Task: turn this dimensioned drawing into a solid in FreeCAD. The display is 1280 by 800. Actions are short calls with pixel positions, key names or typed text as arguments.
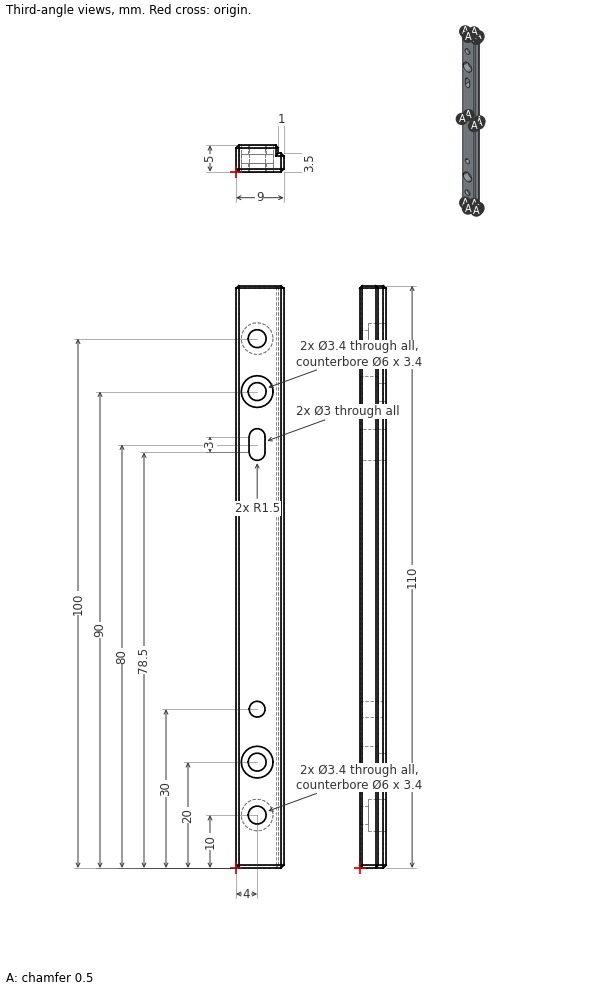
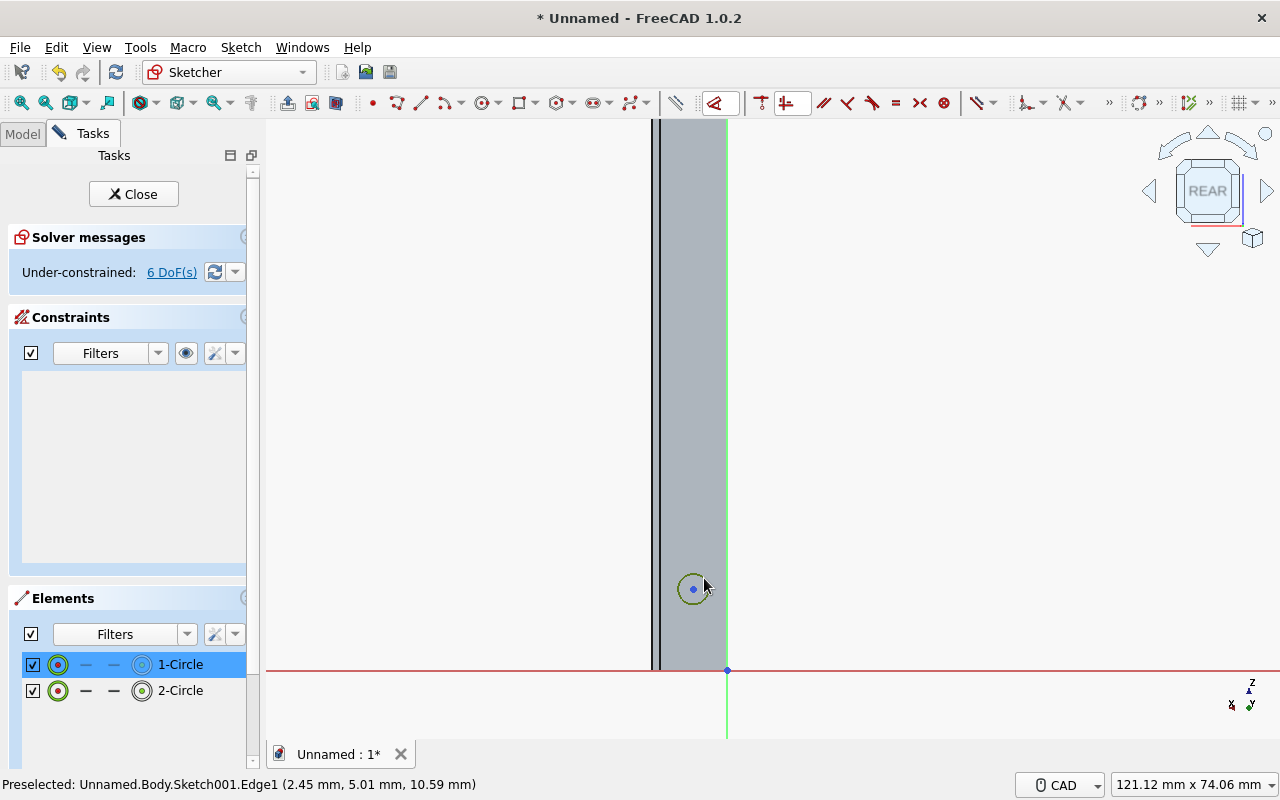
scroll(706, 579, down, 4)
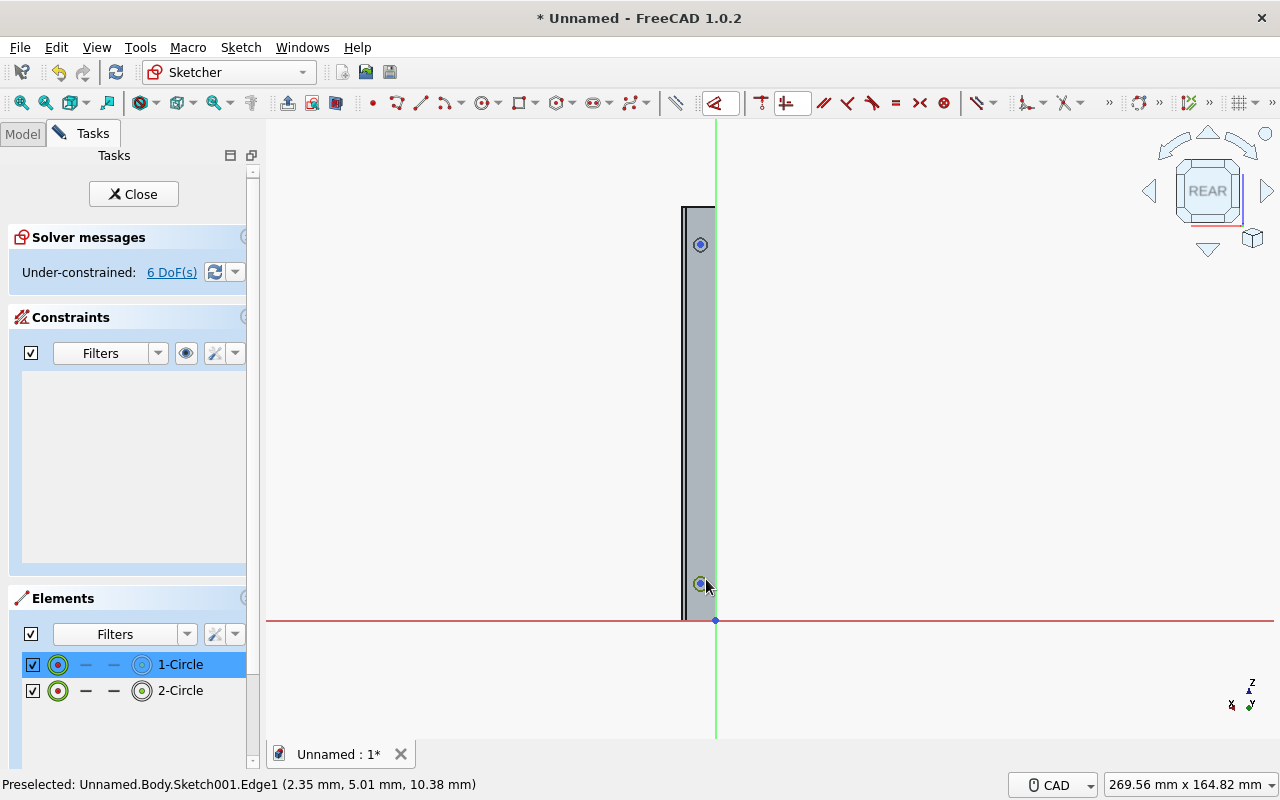
scroll(705, 240, up, 4)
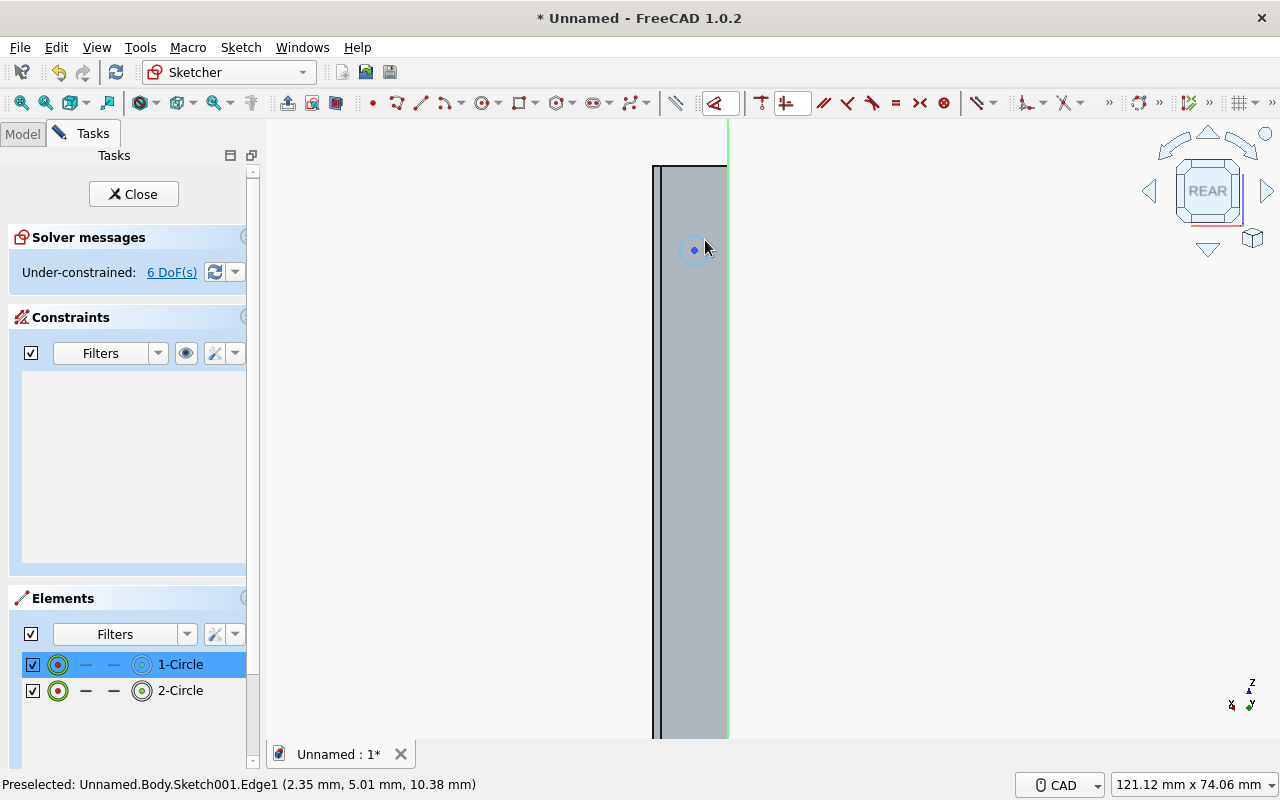
click(705, 240)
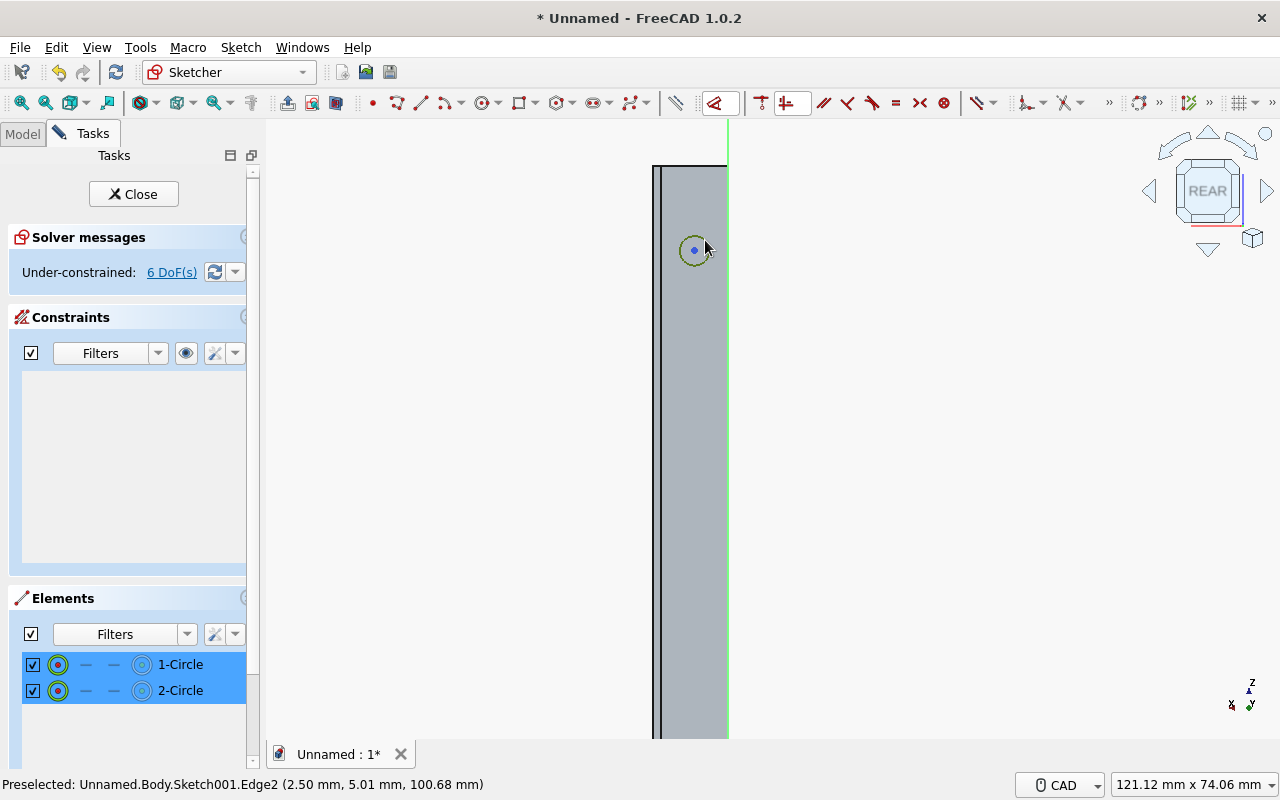
key(e)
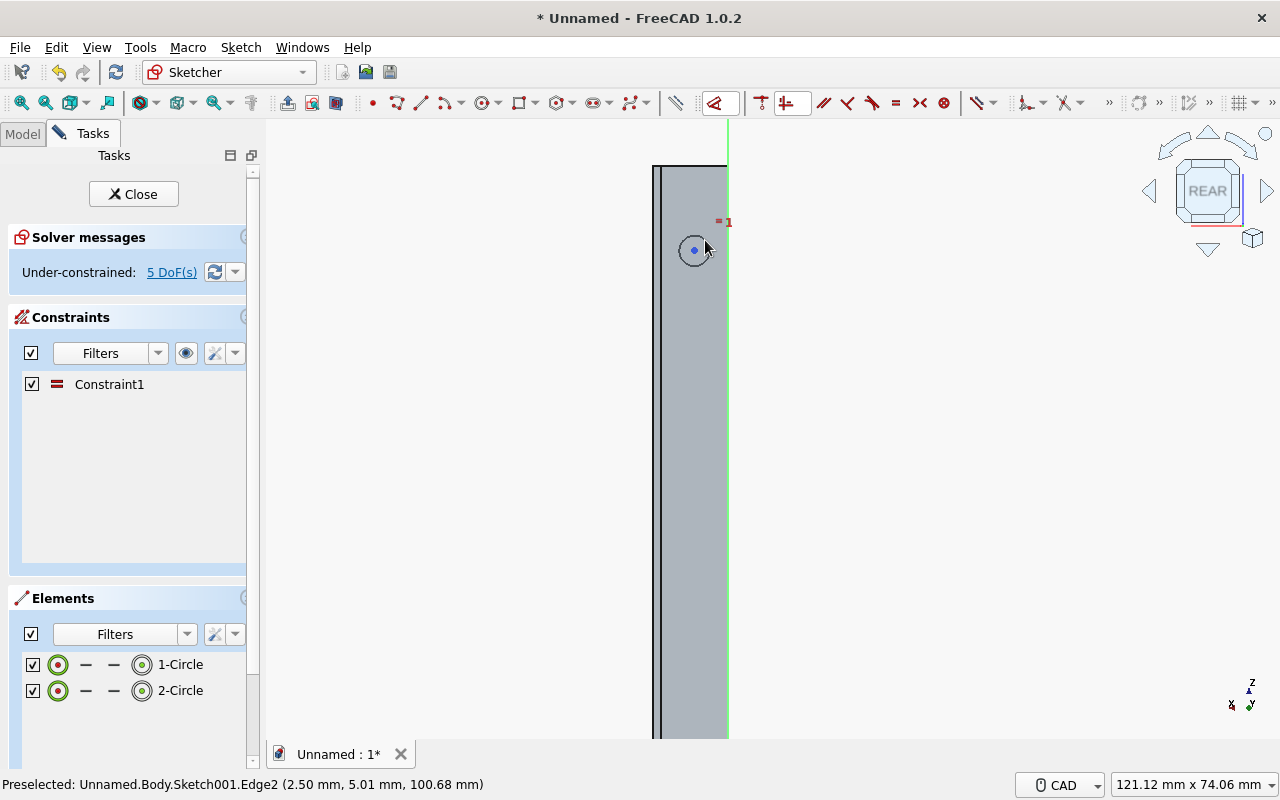
key(d)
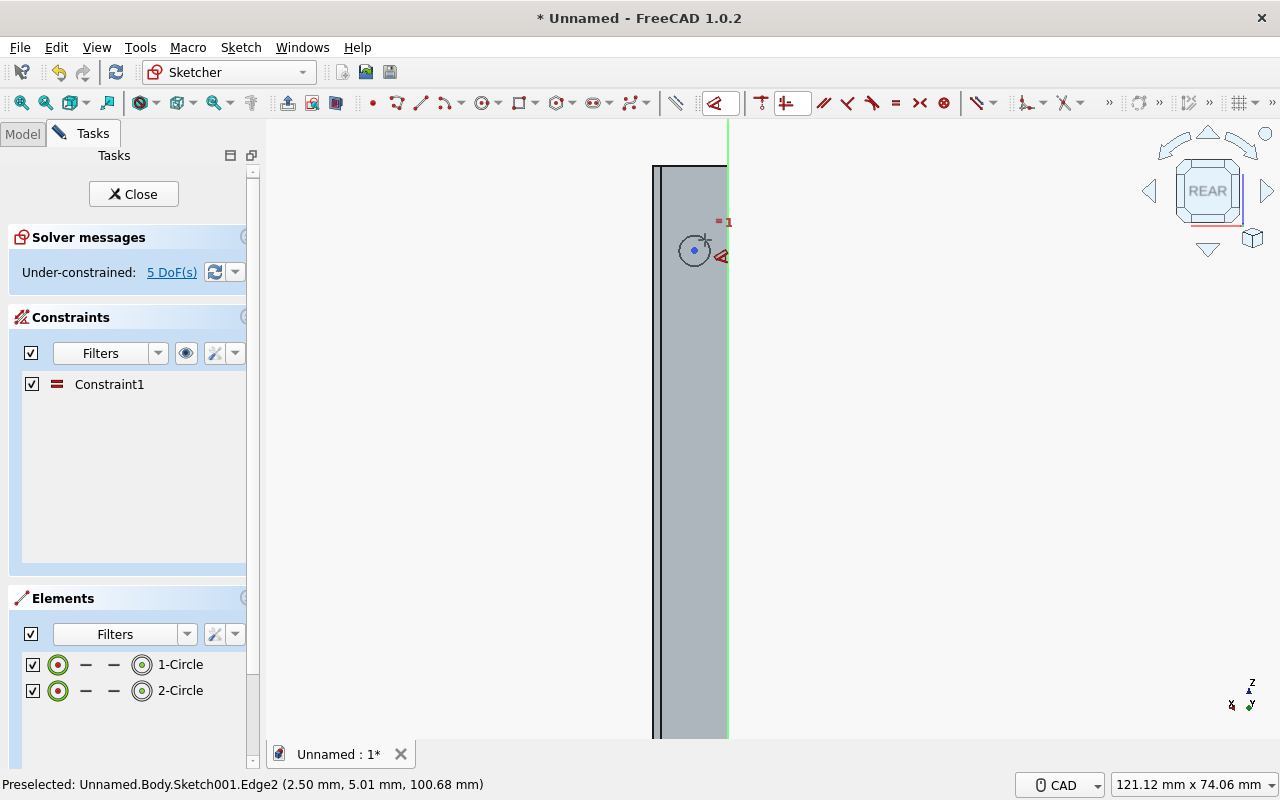
scroll(705, 240, down, 4)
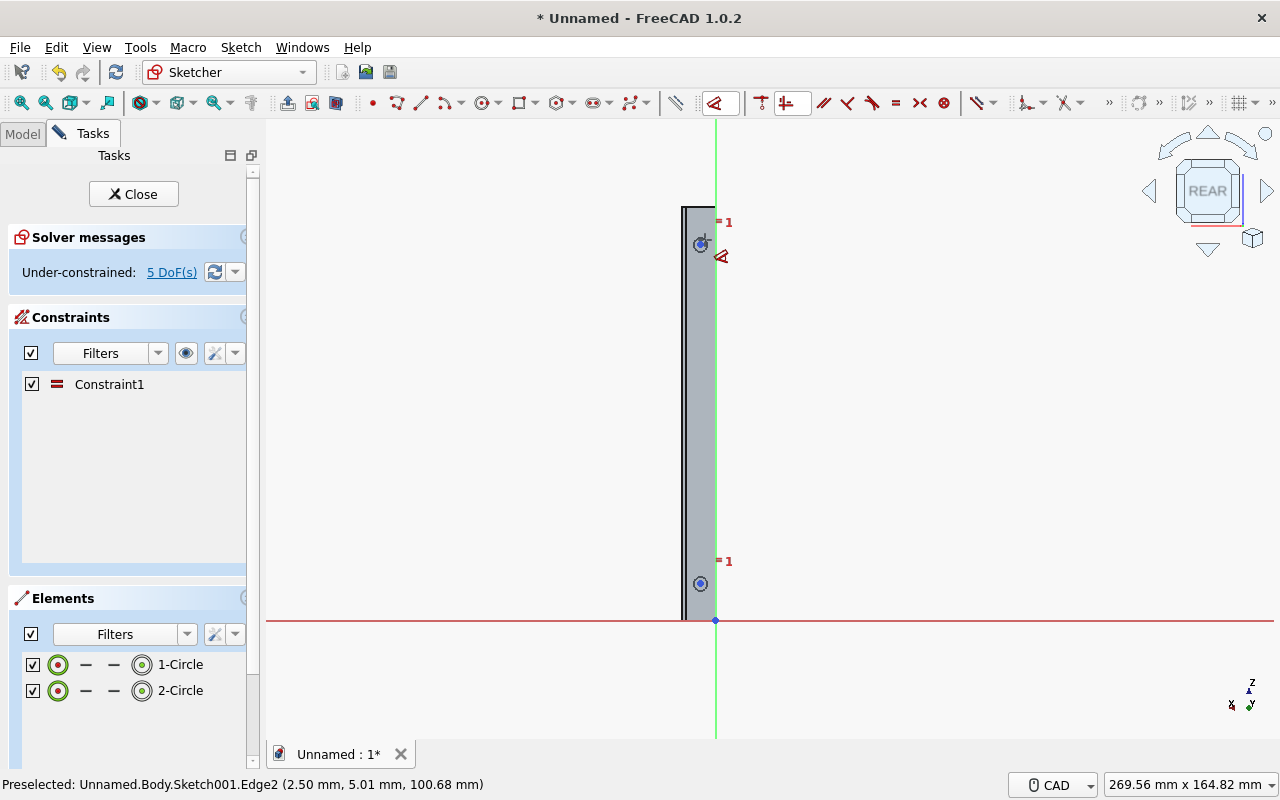
scroll(705, 579, up, 6)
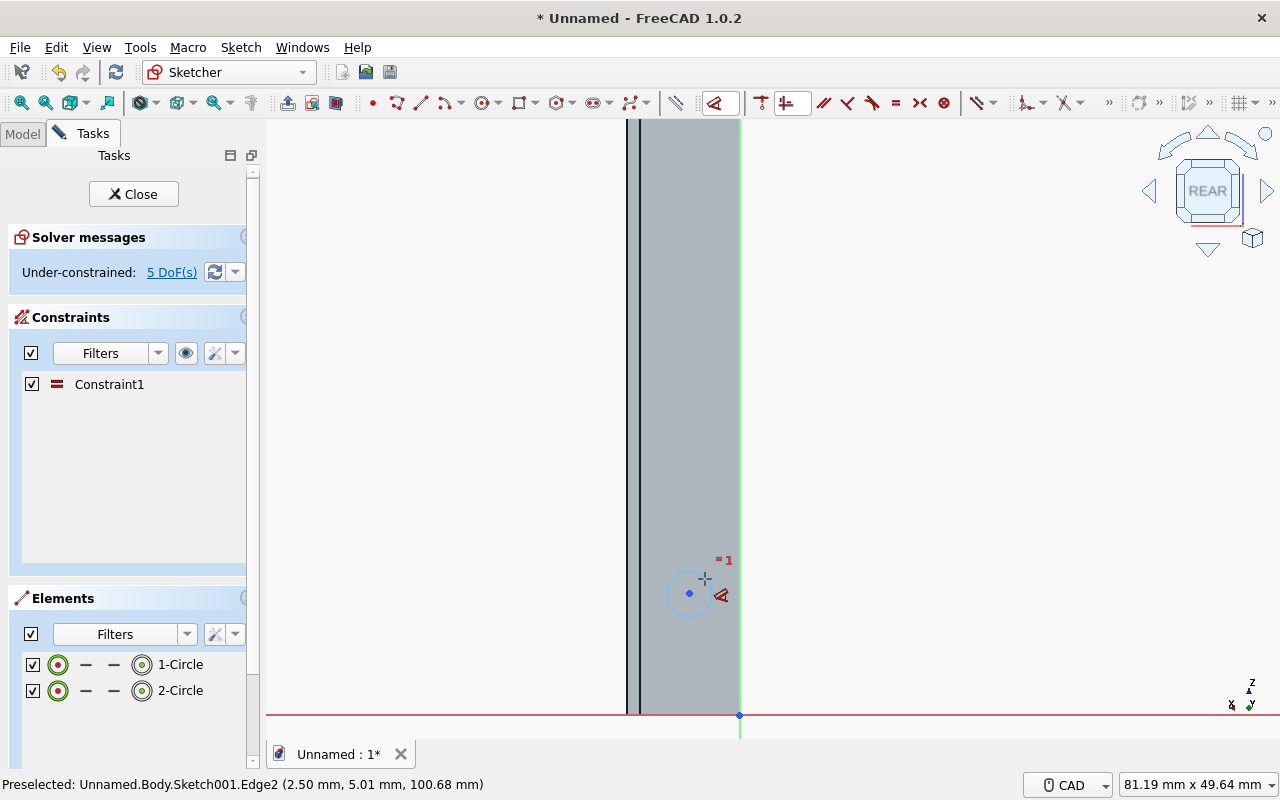
click(705, 578)
click(704, 542)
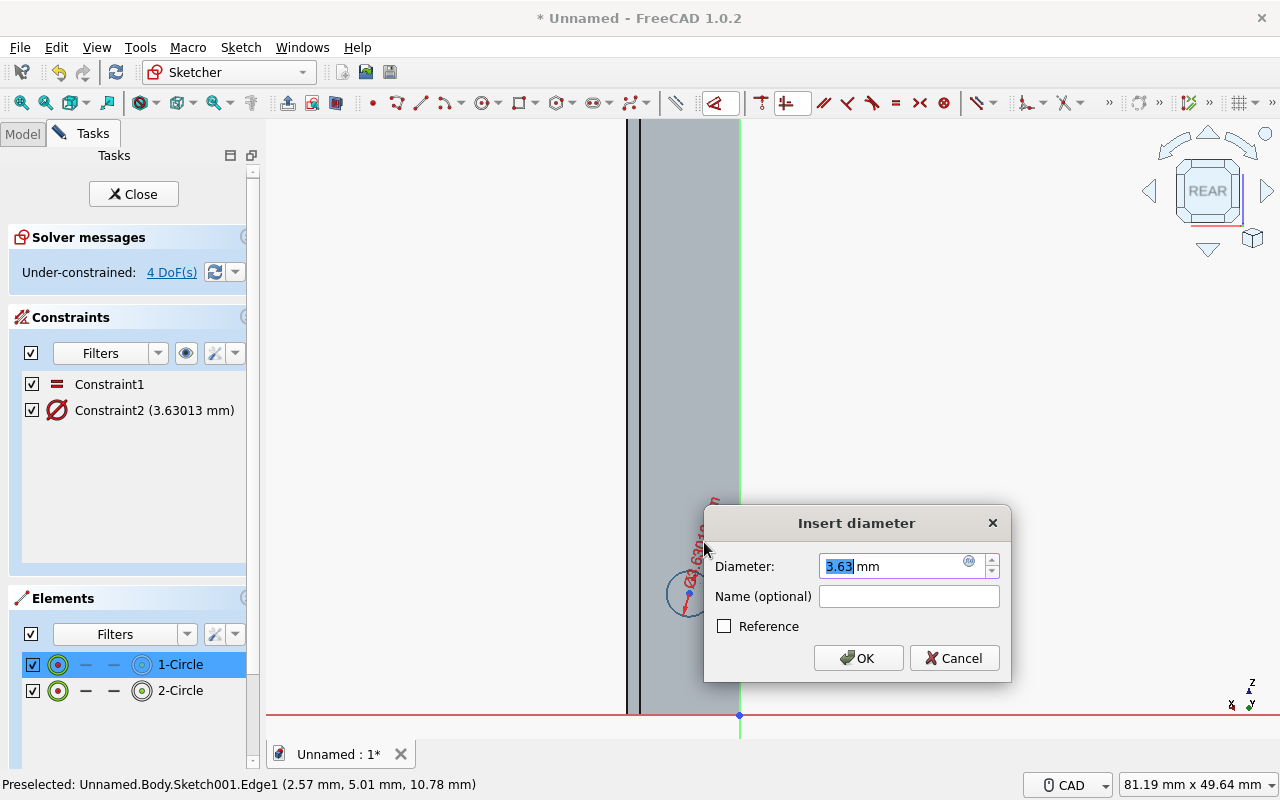
text(3.4)
key(Return)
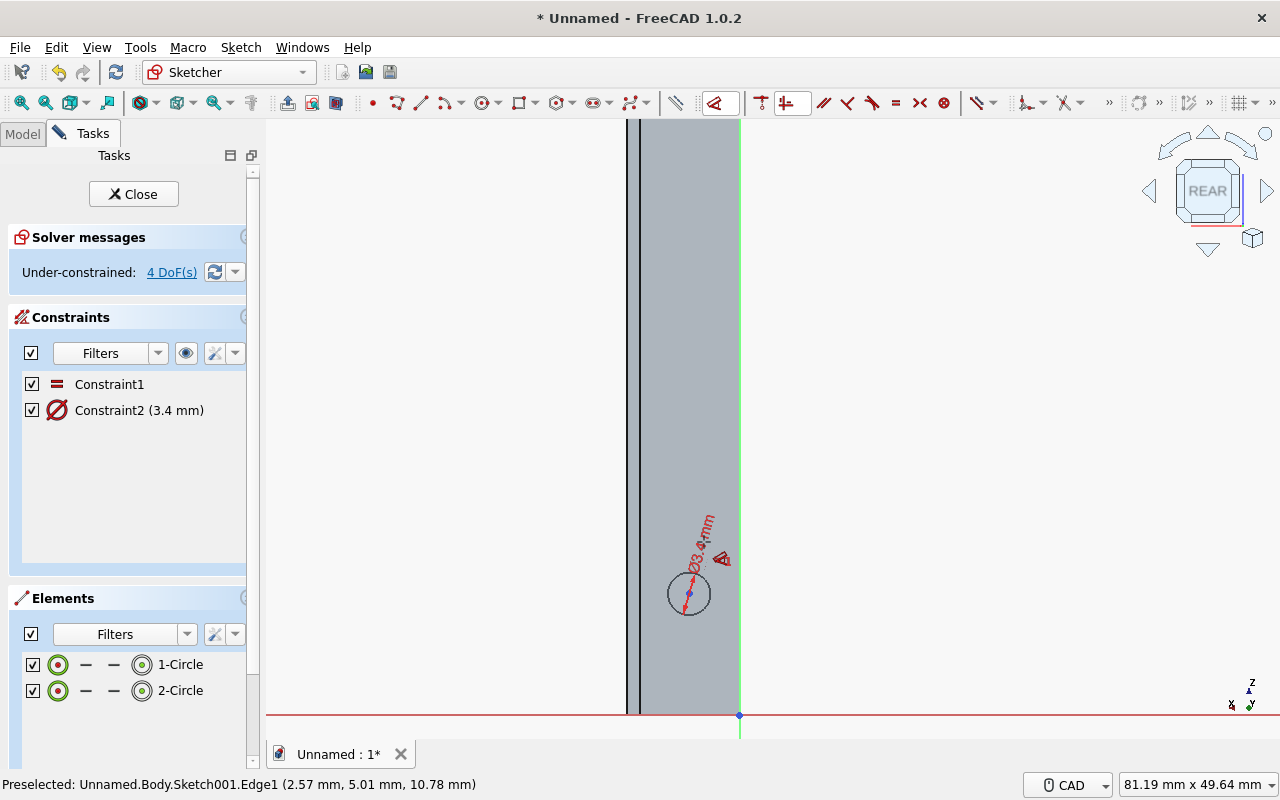
click(689, 594)
click(714, 512)